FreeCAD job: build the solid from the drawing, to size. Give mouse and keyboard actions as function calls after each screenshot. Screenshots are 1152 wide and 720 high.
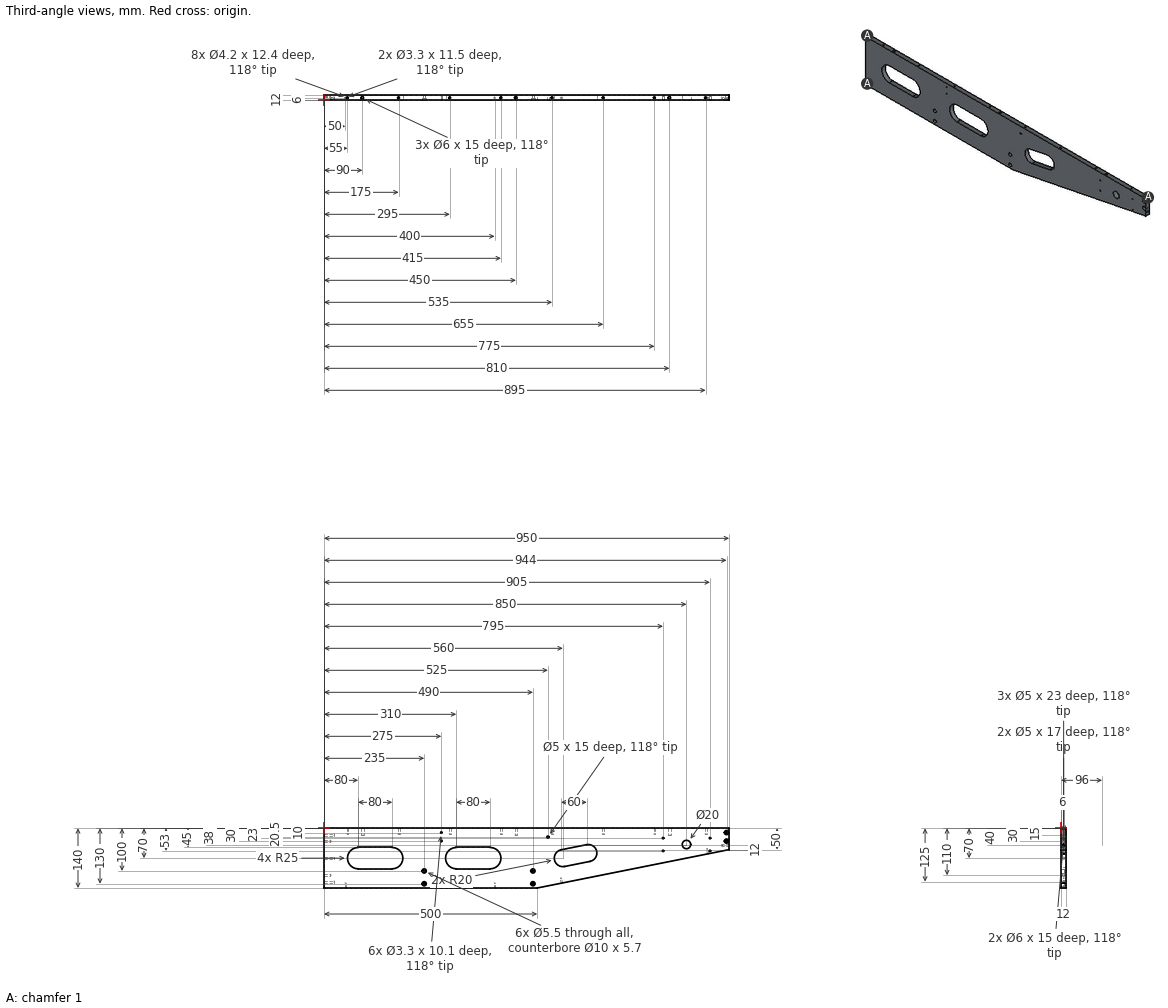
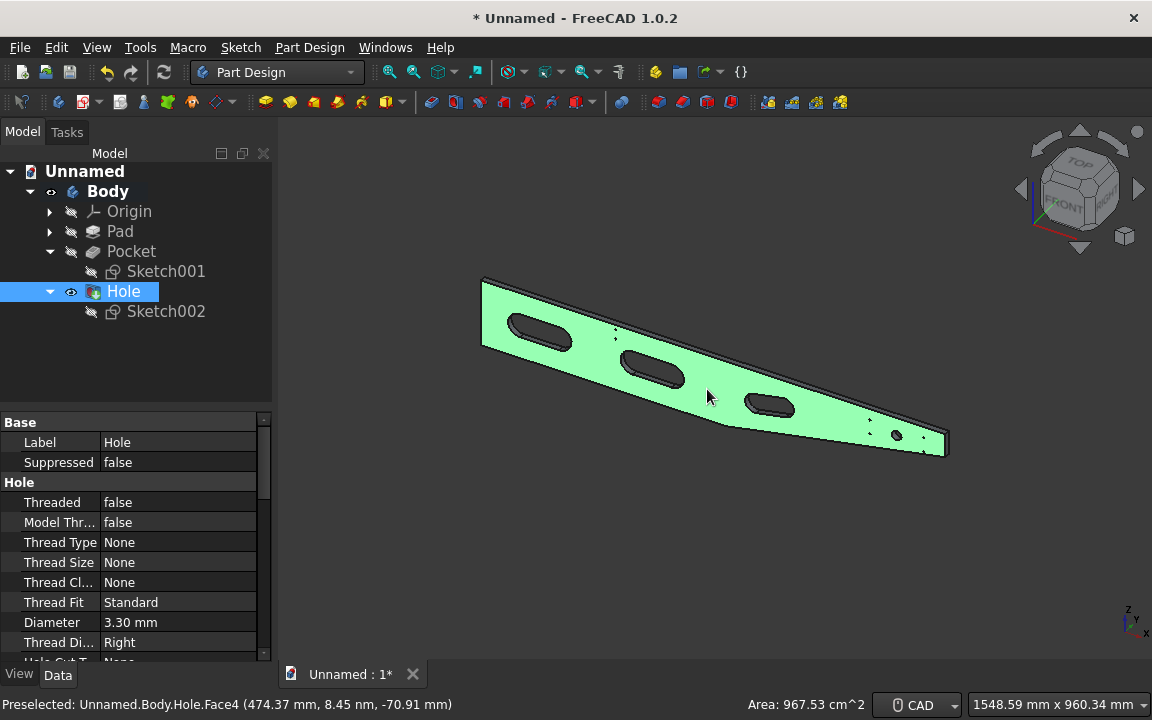
click(84, 102)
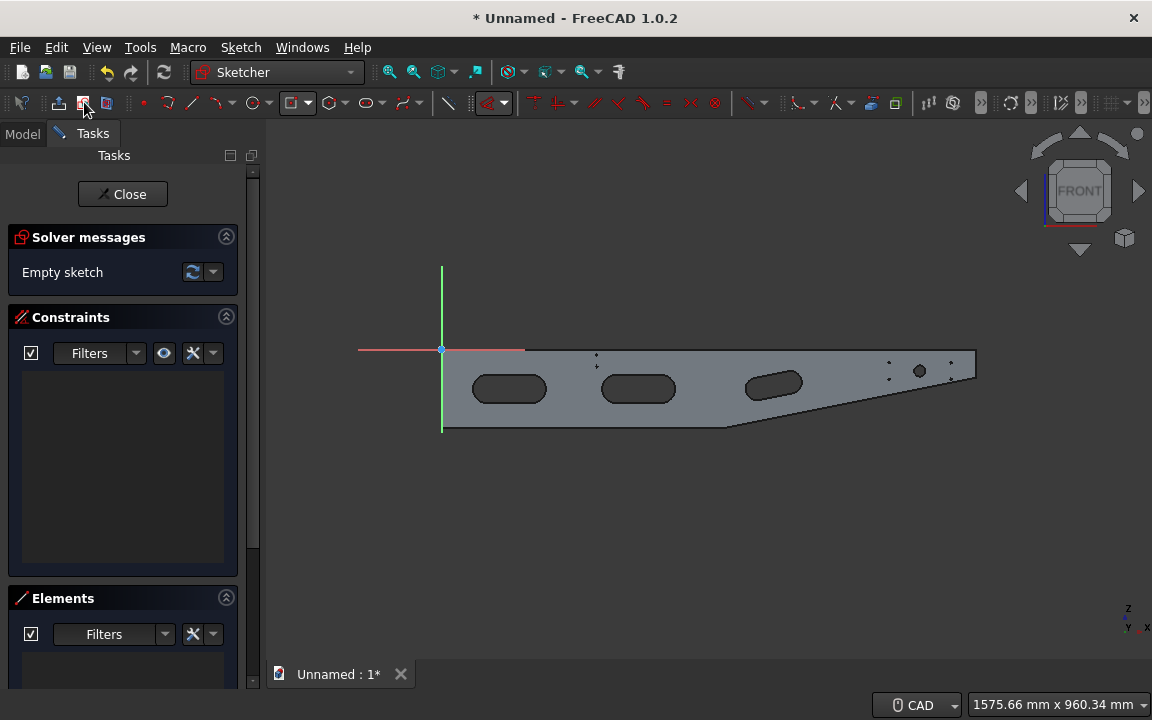
scroll(742, 360, up, 15)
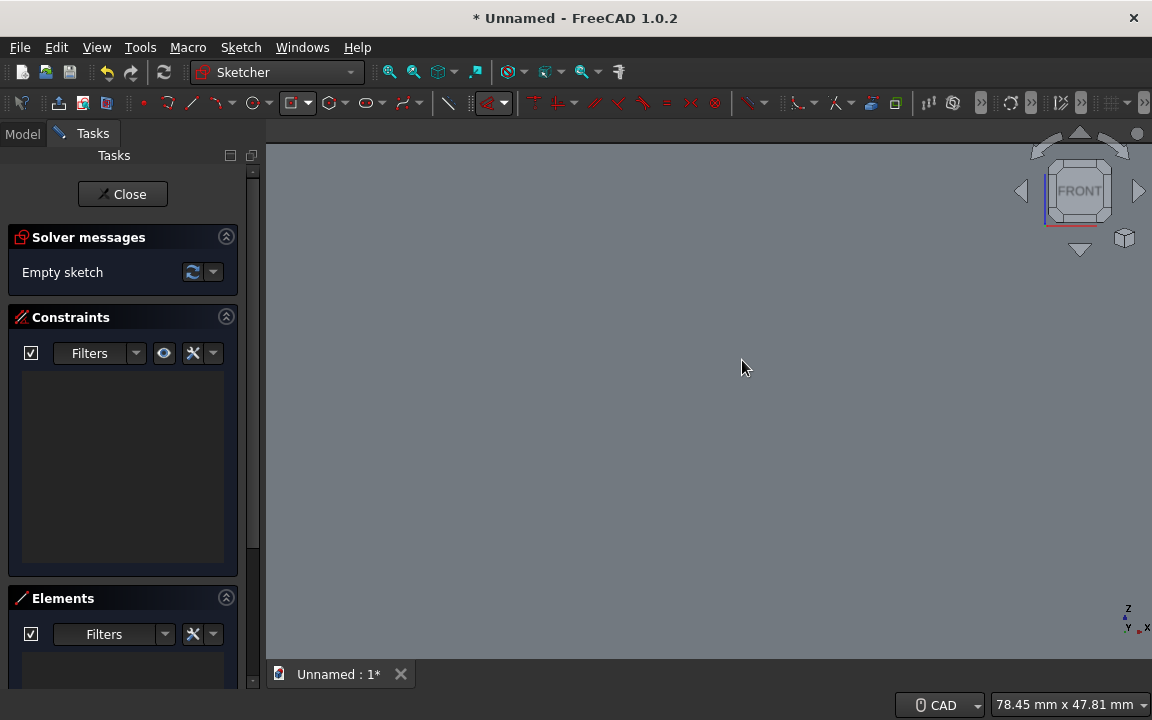
scroll(632, 372, up, 9)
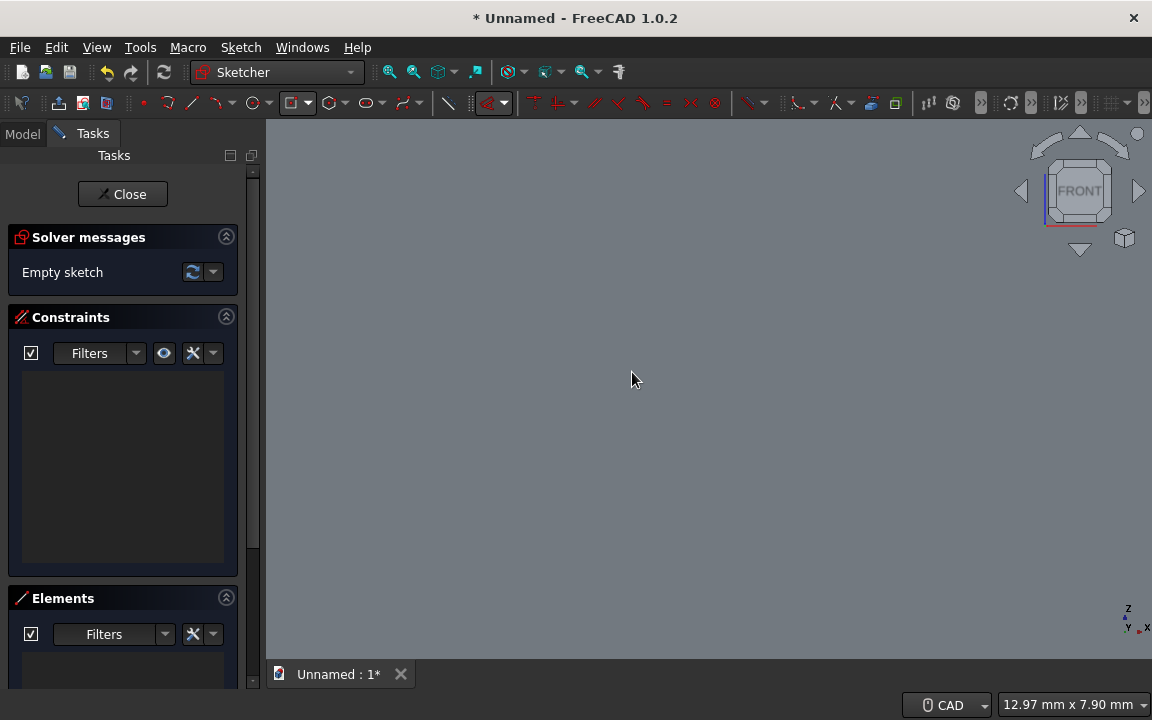
click(254, 104)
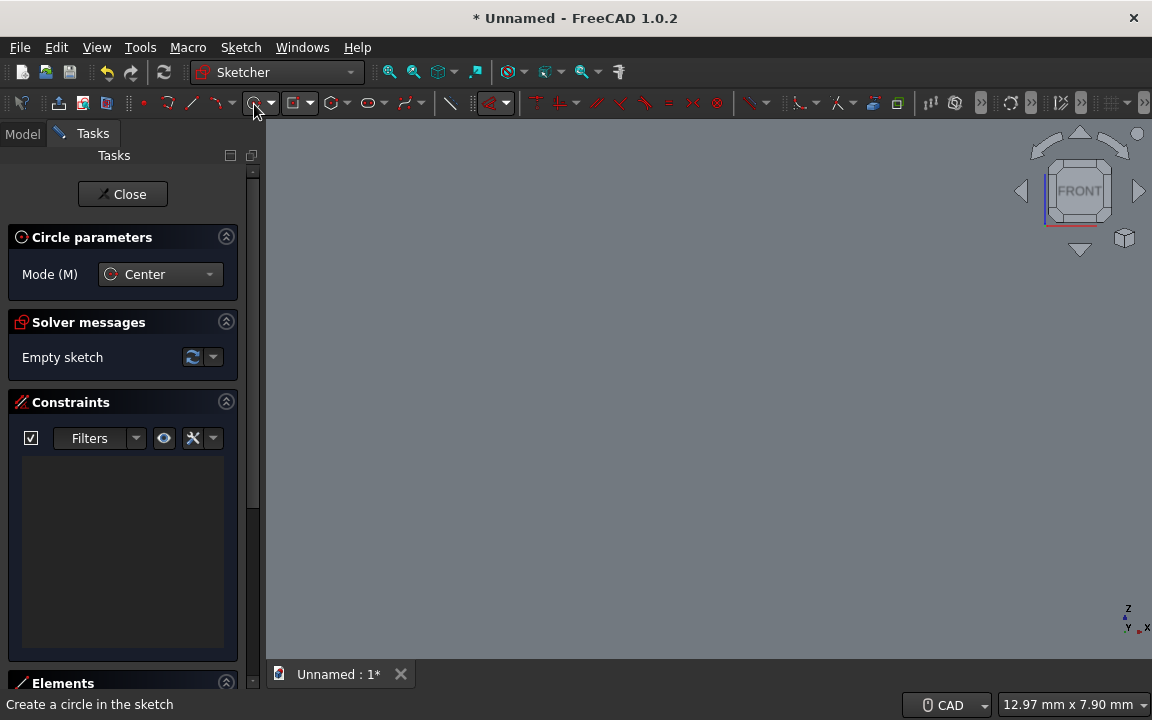
click(640, 387)
move(760, 266)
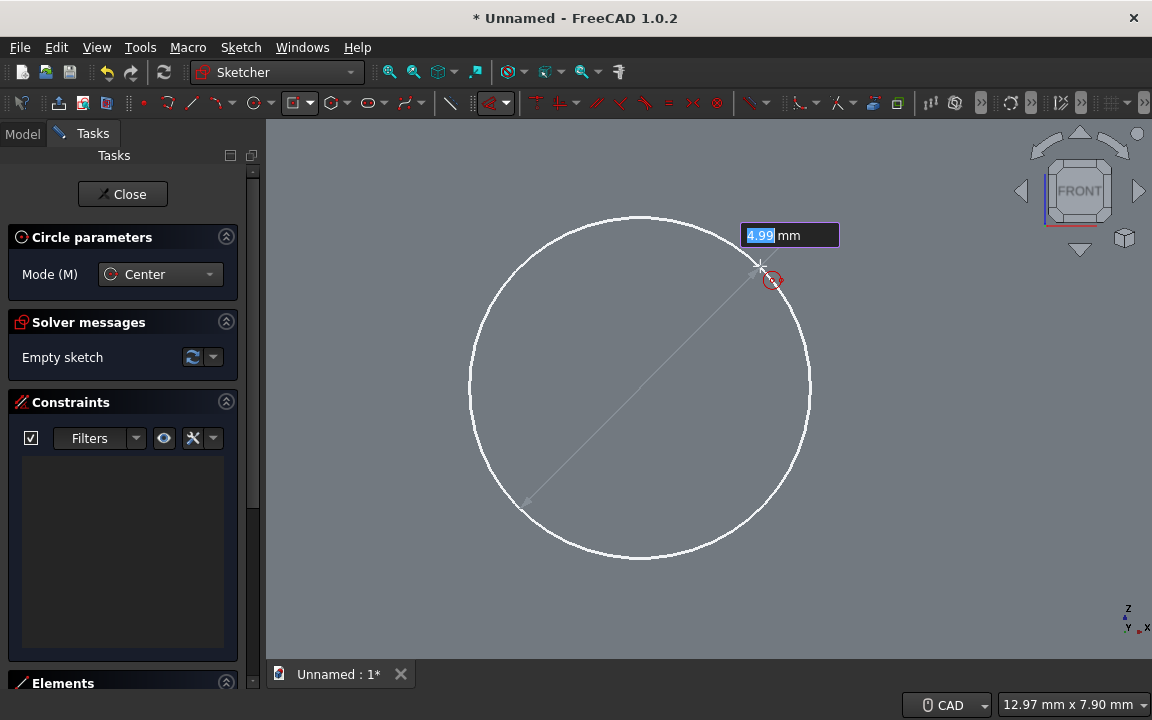
text(5)
key(Return)
key(Escape)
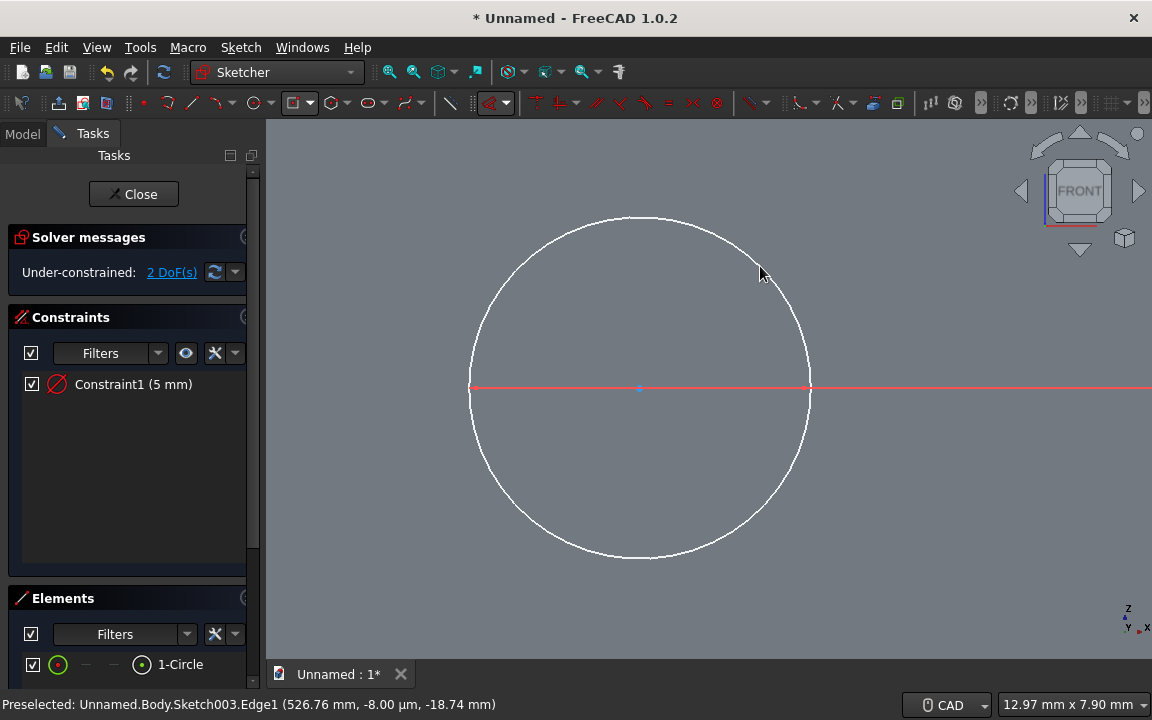
click(640, 388)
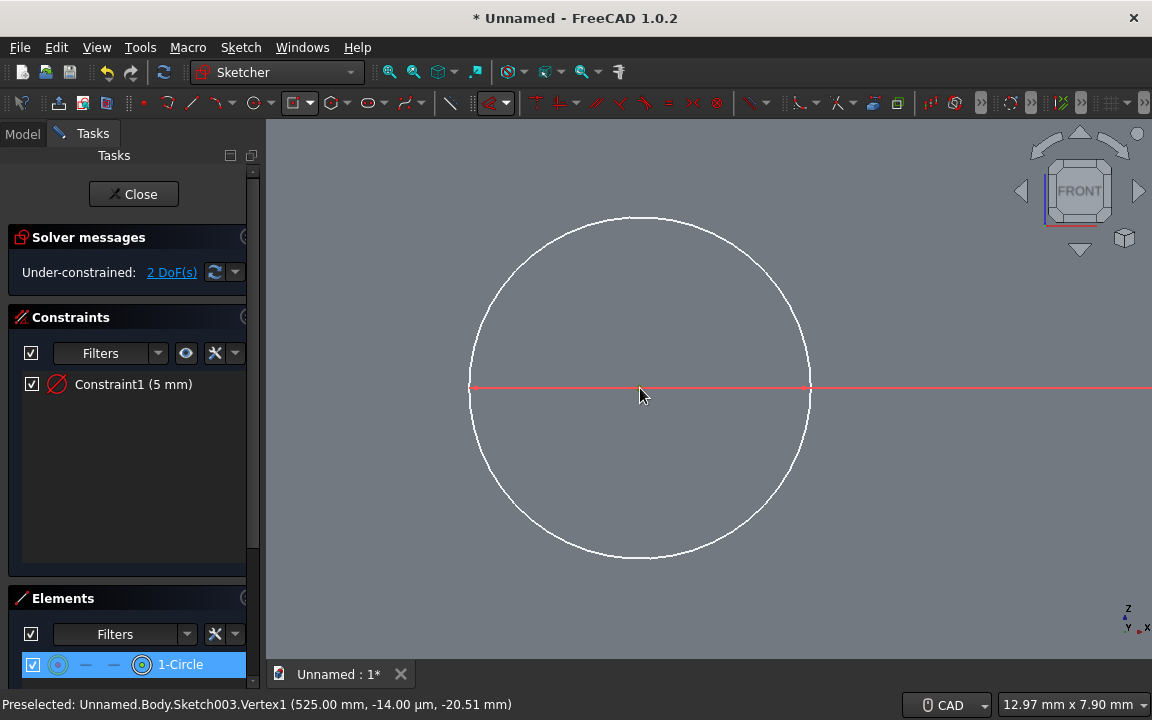
key(l)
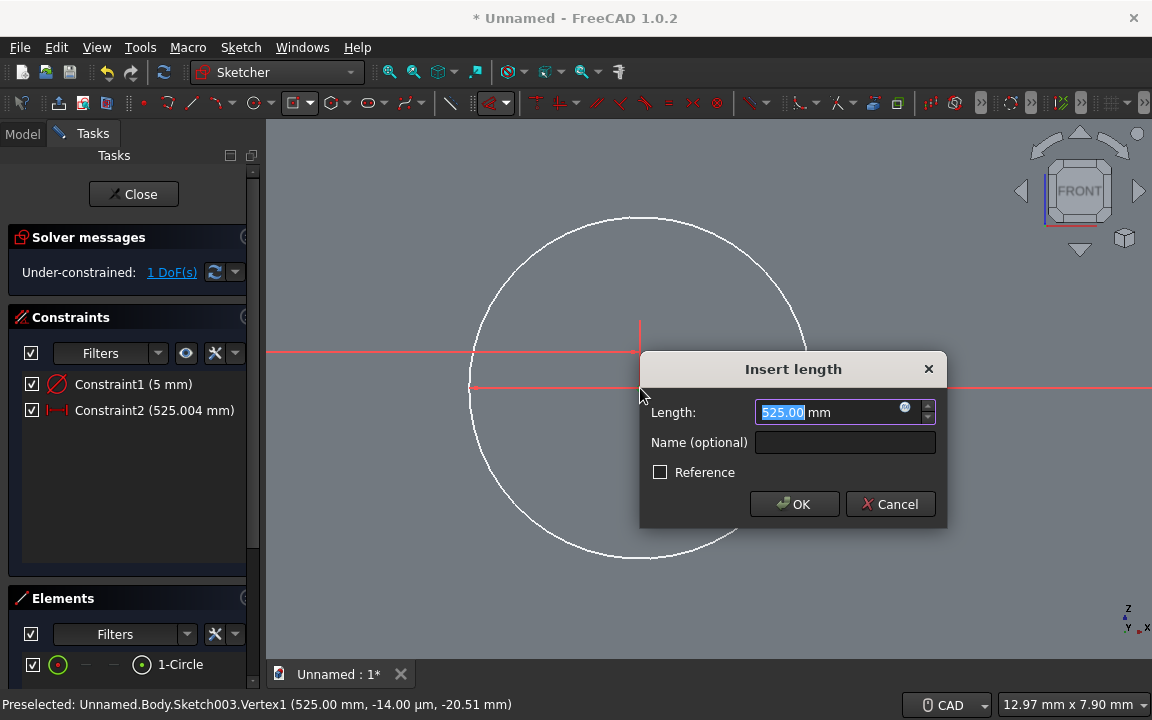
text(525)
key(Return)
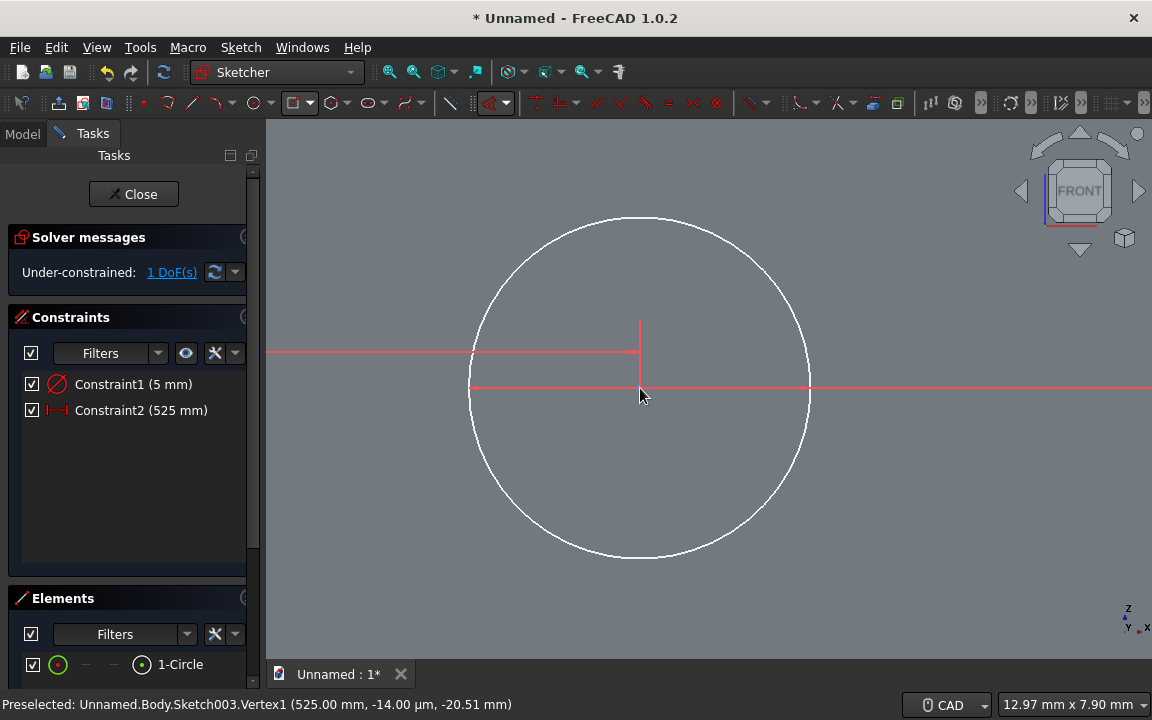
click(640, 388)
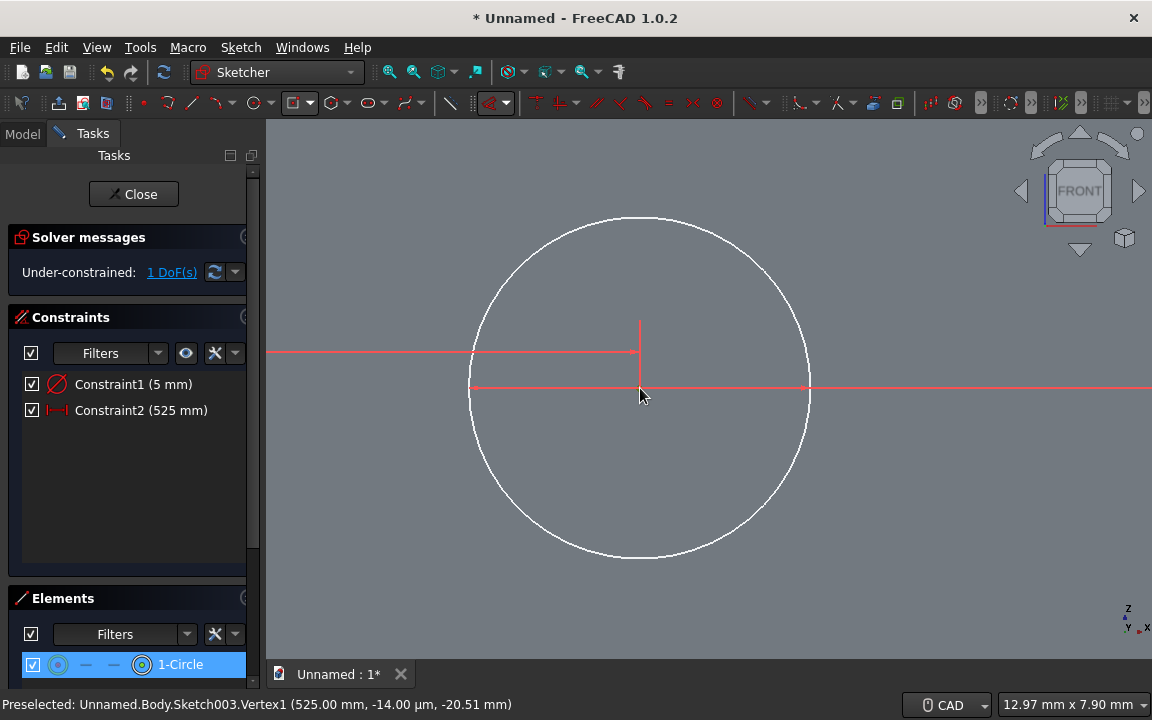
key(i)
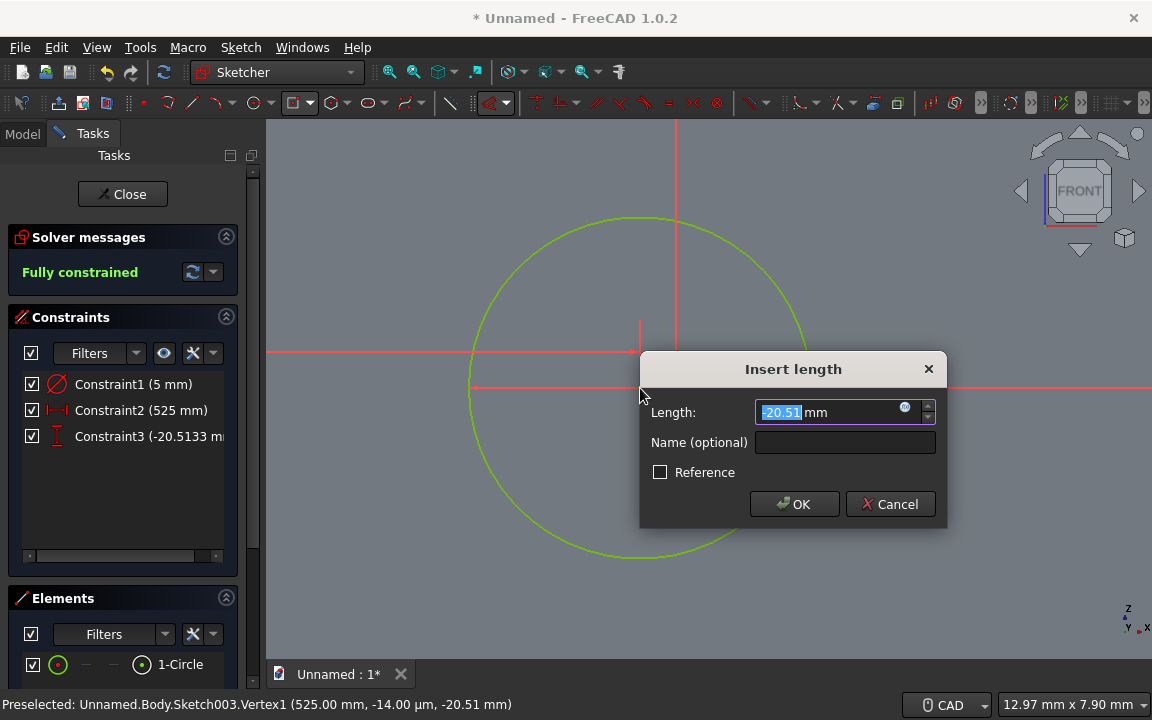
text(-20.5)
key(Return)